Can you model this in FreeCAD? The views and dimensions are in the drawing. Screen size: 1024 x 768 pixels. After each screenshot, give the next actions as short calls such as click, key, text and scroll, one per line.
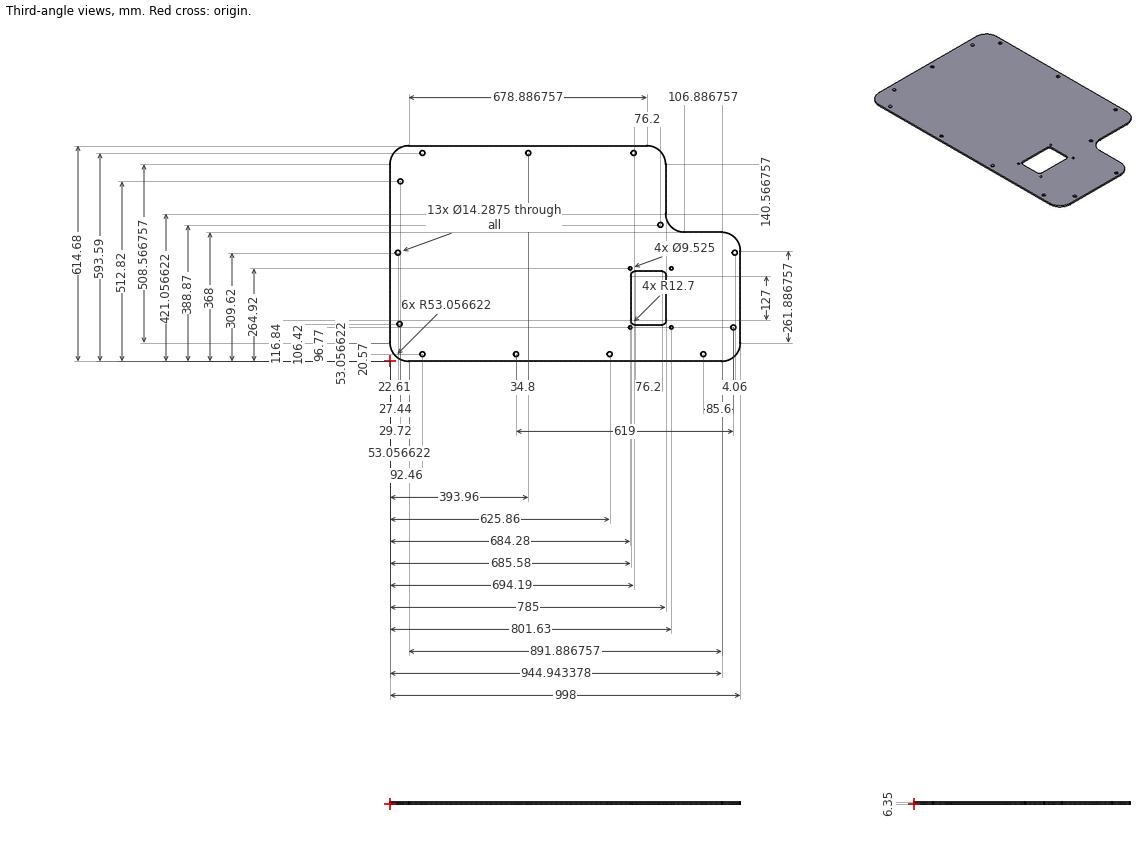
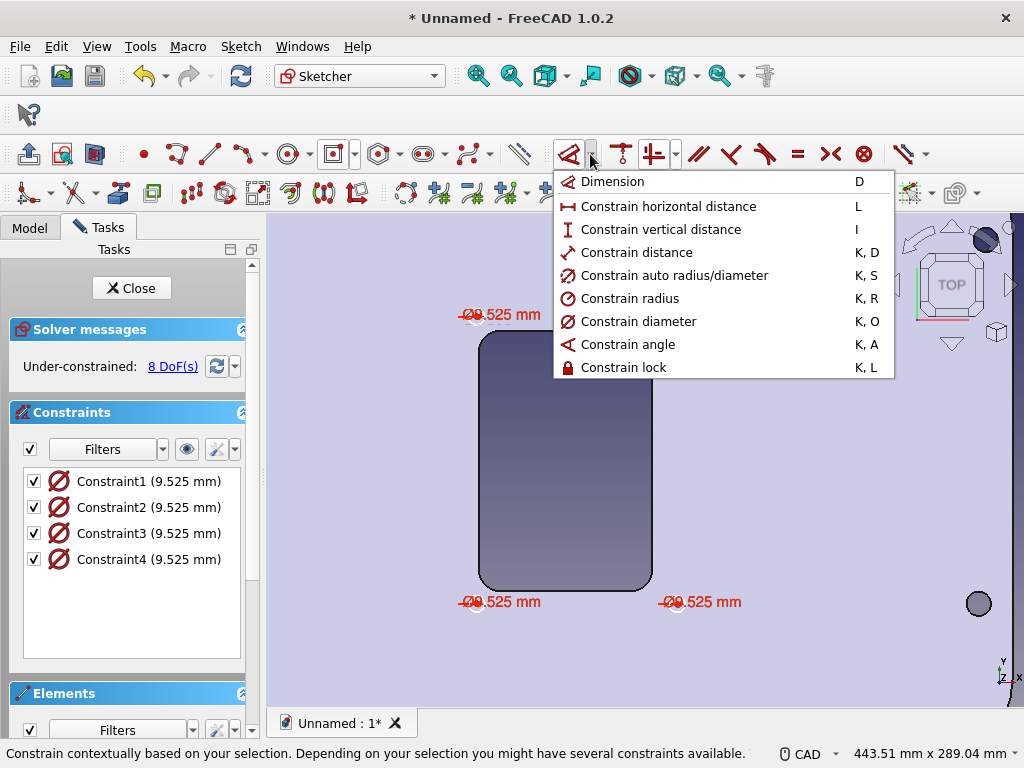
click(724, 230)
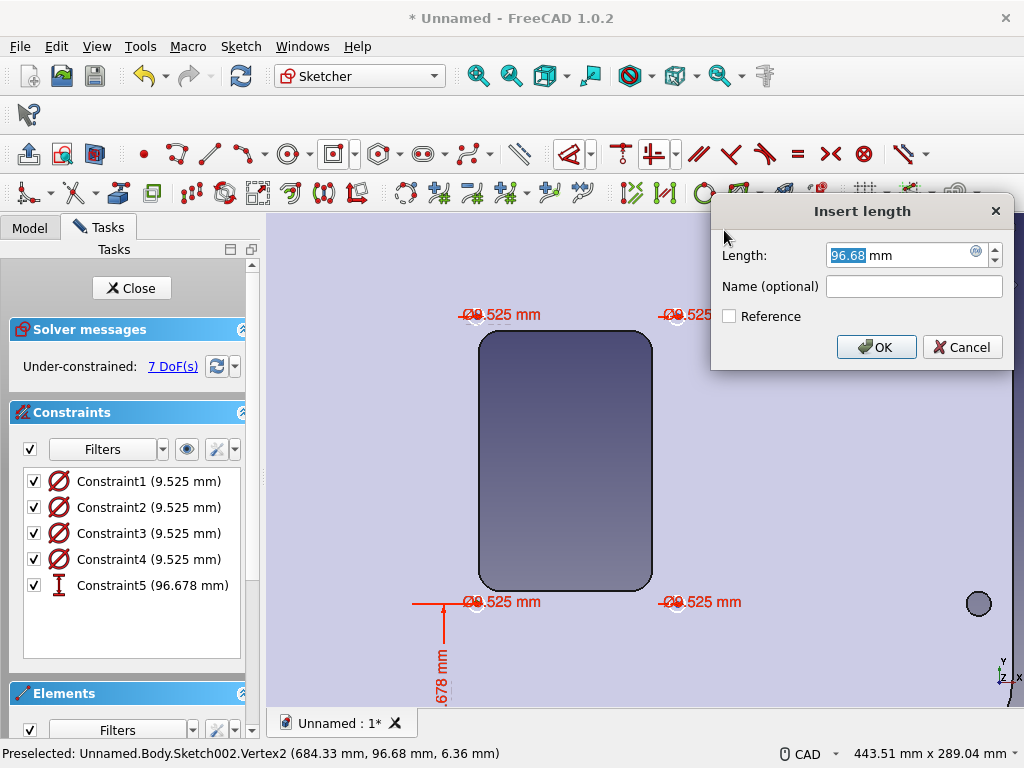
text(96.77)
key(Return)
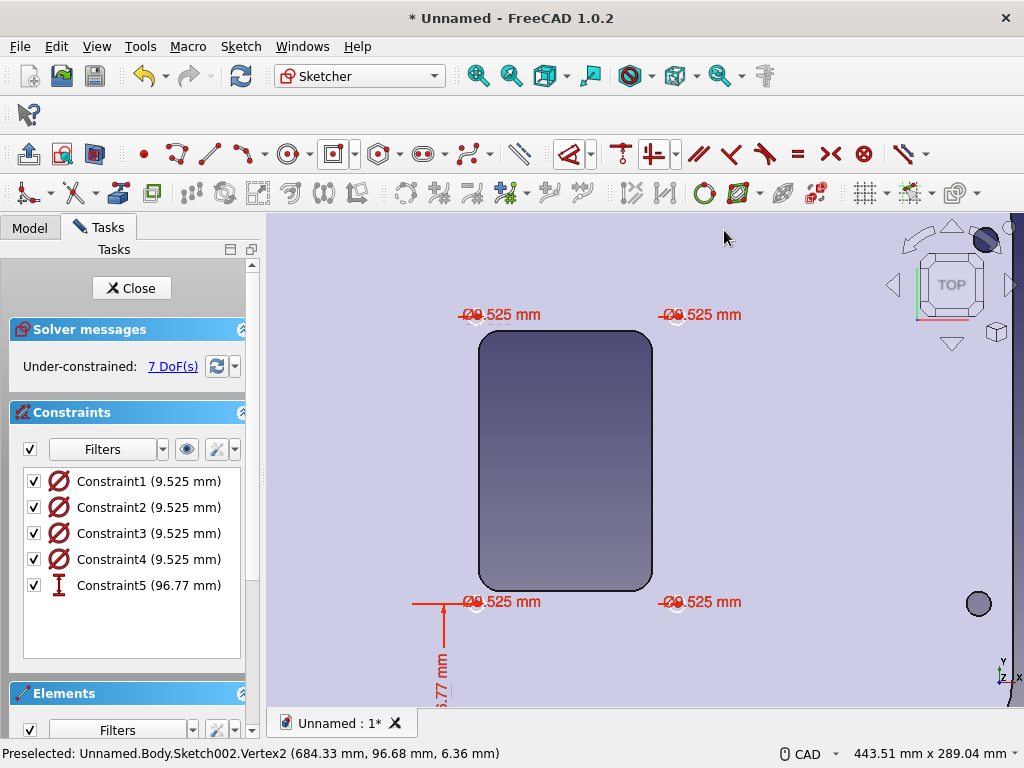
click(677, 604)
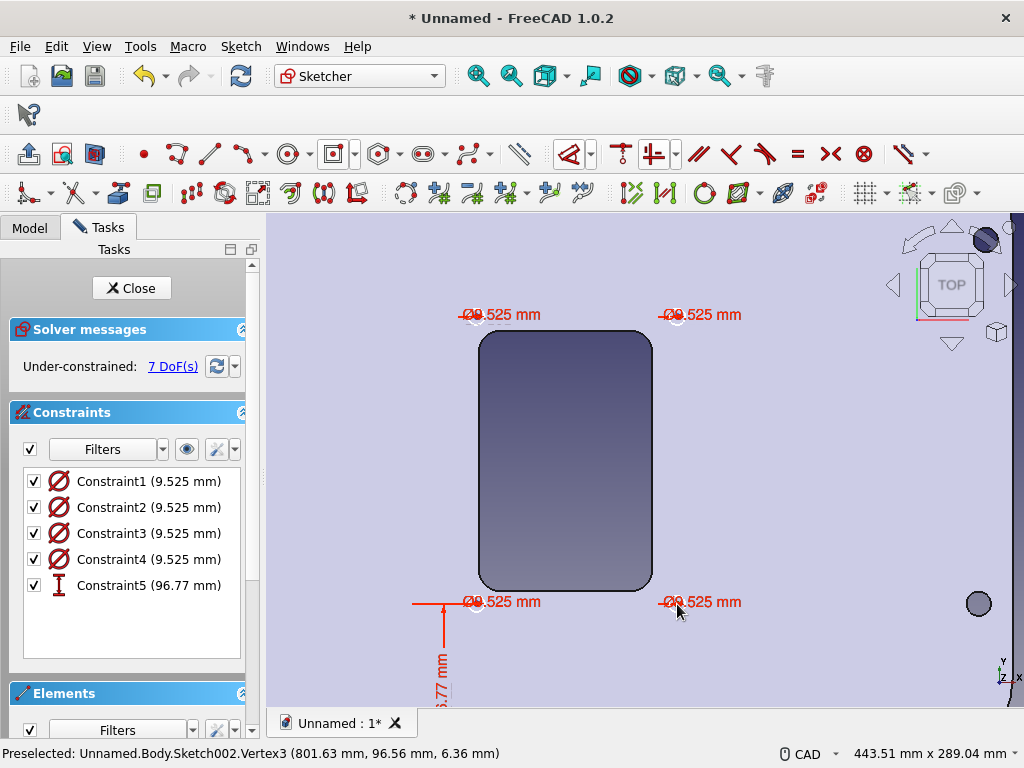
click(590, 154)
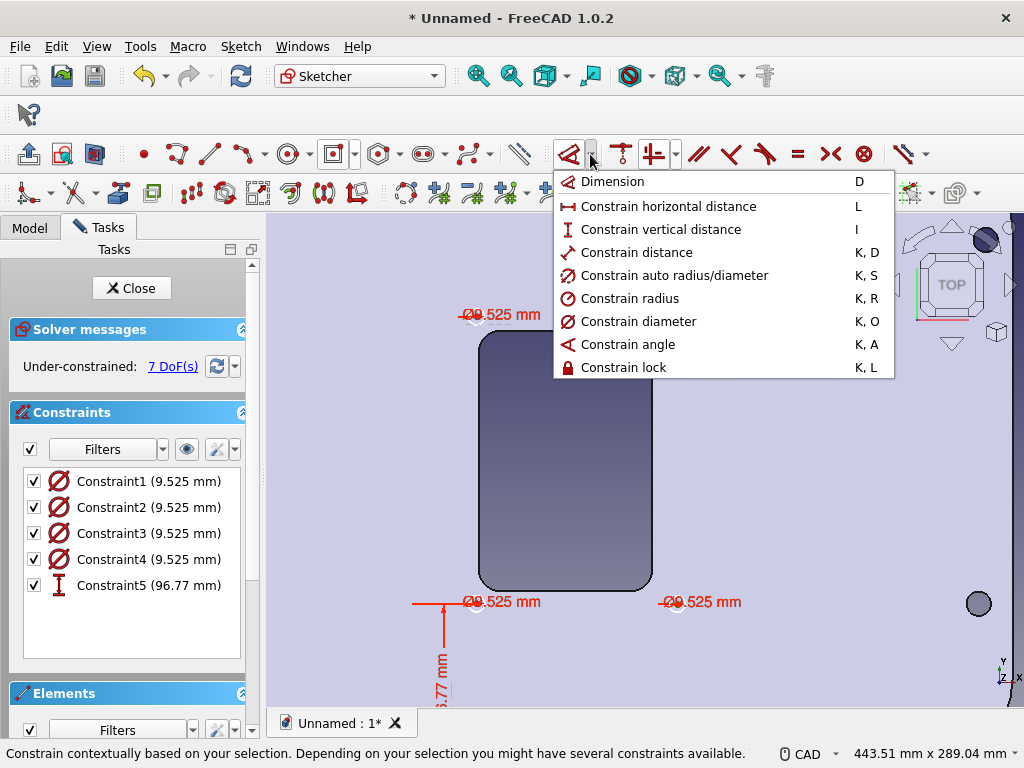
click(724, 230)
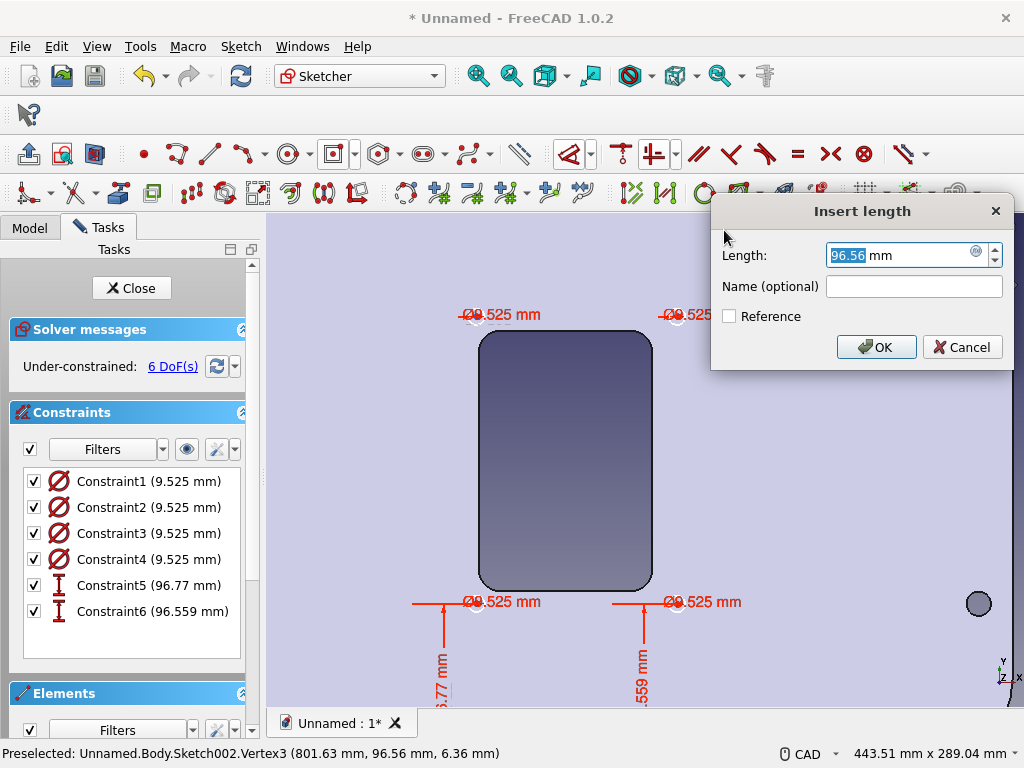
text(96.77)
key(Return)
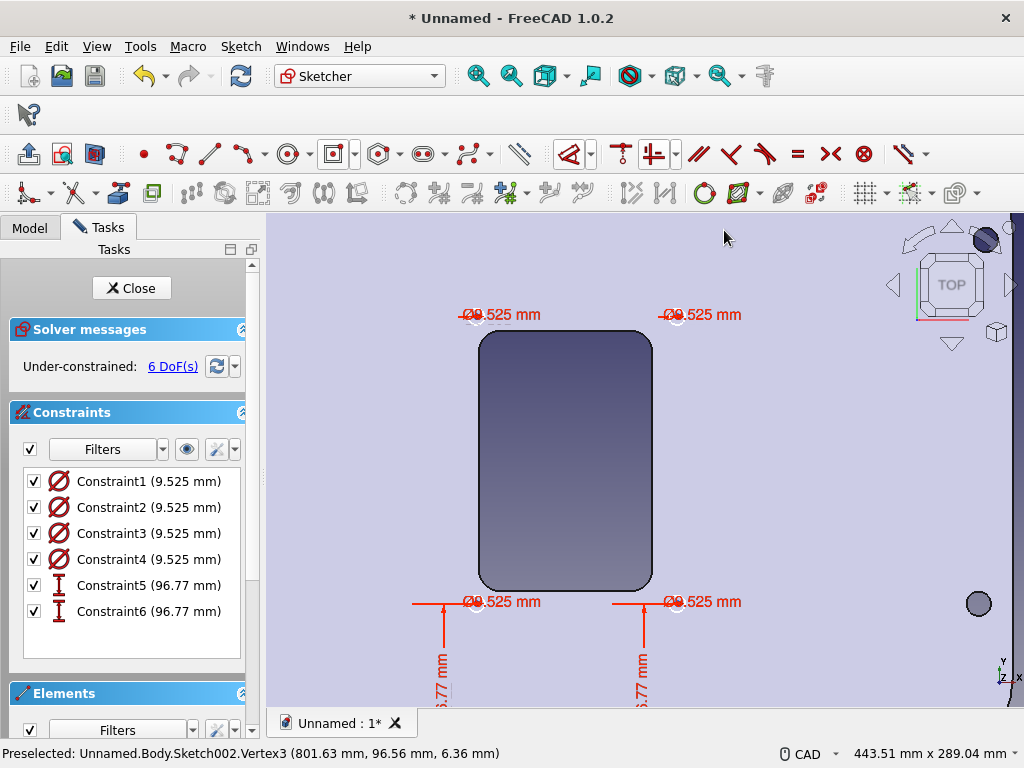
click(476, 317)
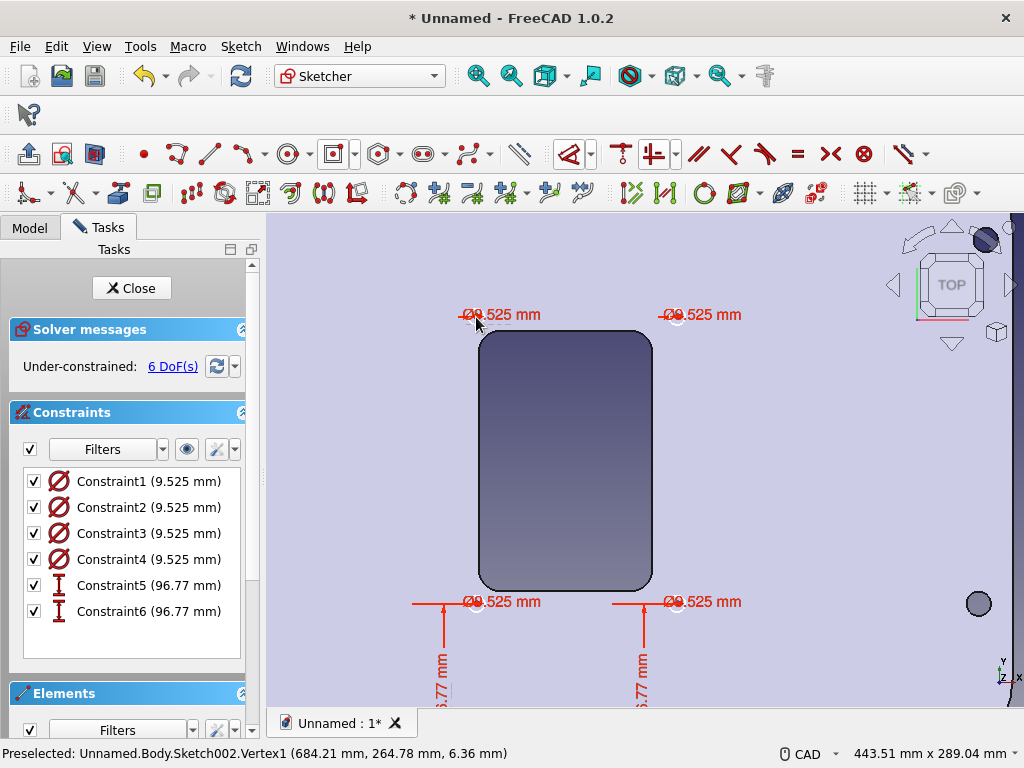
key(l)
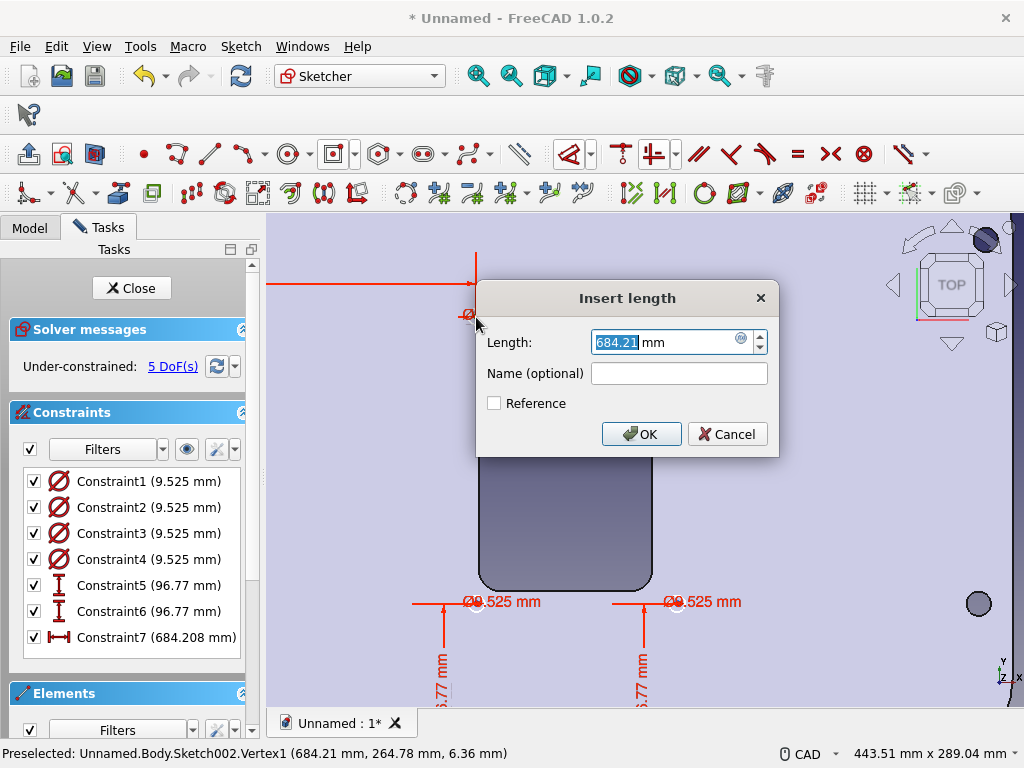
text(684.28)
key(Return)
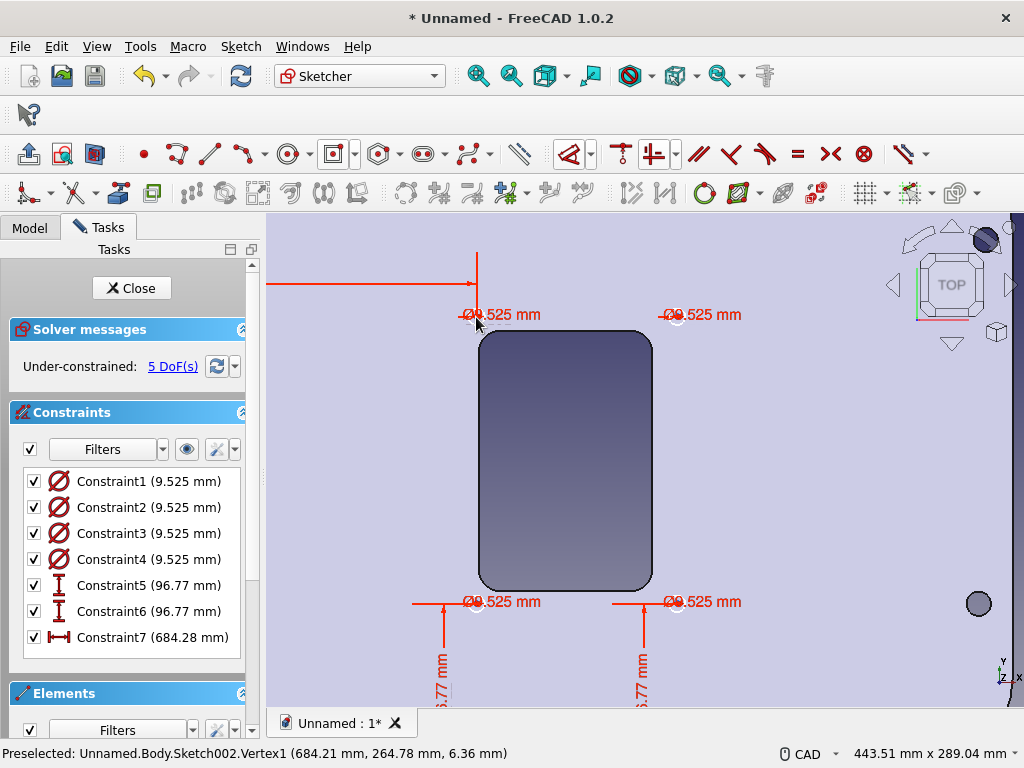
click(477, 317)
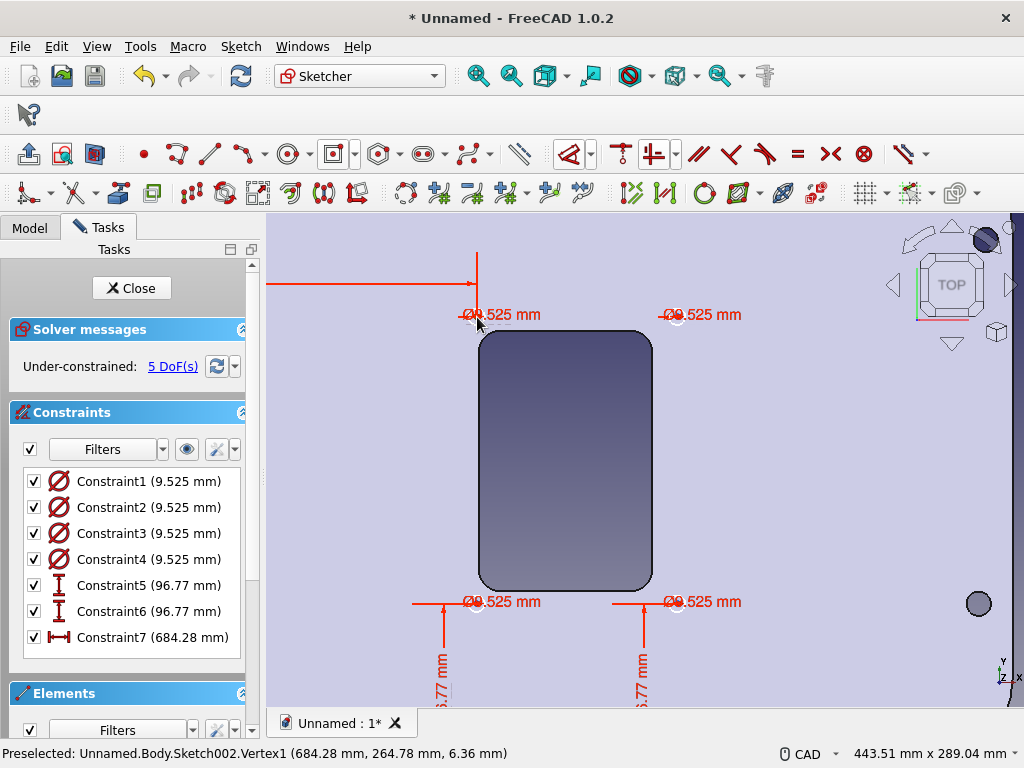
click(590, 154)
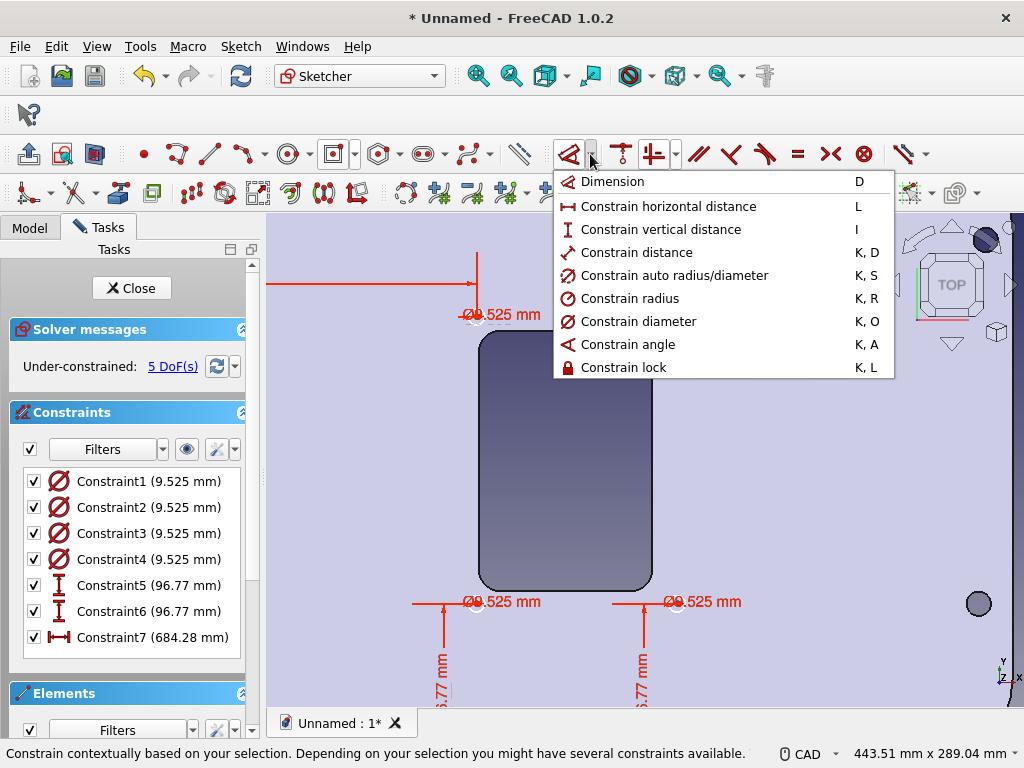
click(724, 230)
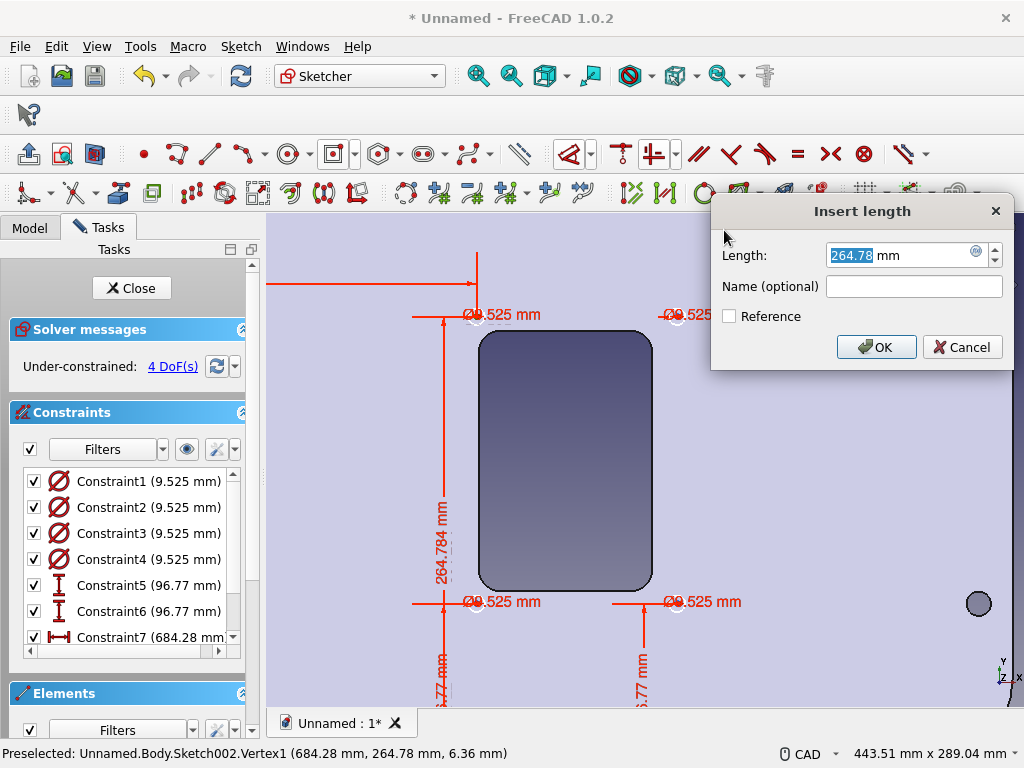
text(264.92)
key(Return)